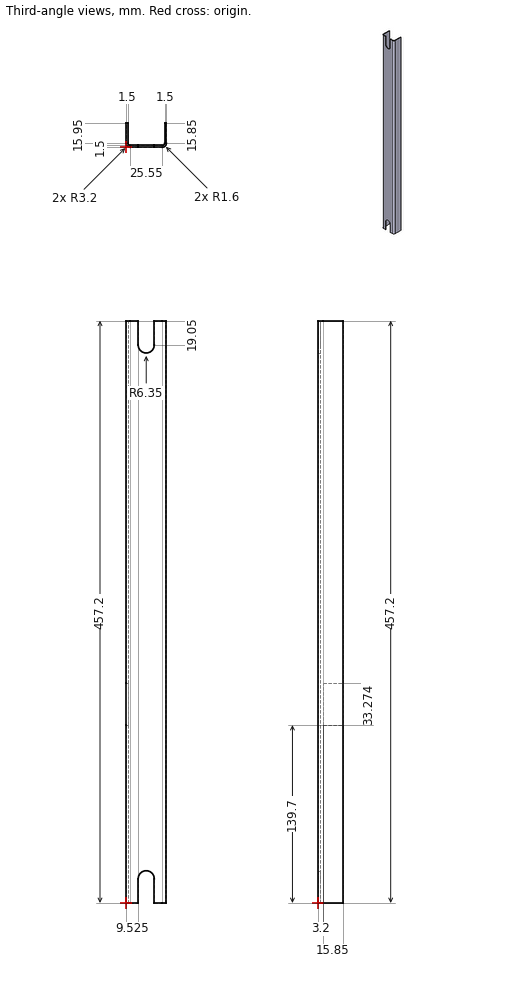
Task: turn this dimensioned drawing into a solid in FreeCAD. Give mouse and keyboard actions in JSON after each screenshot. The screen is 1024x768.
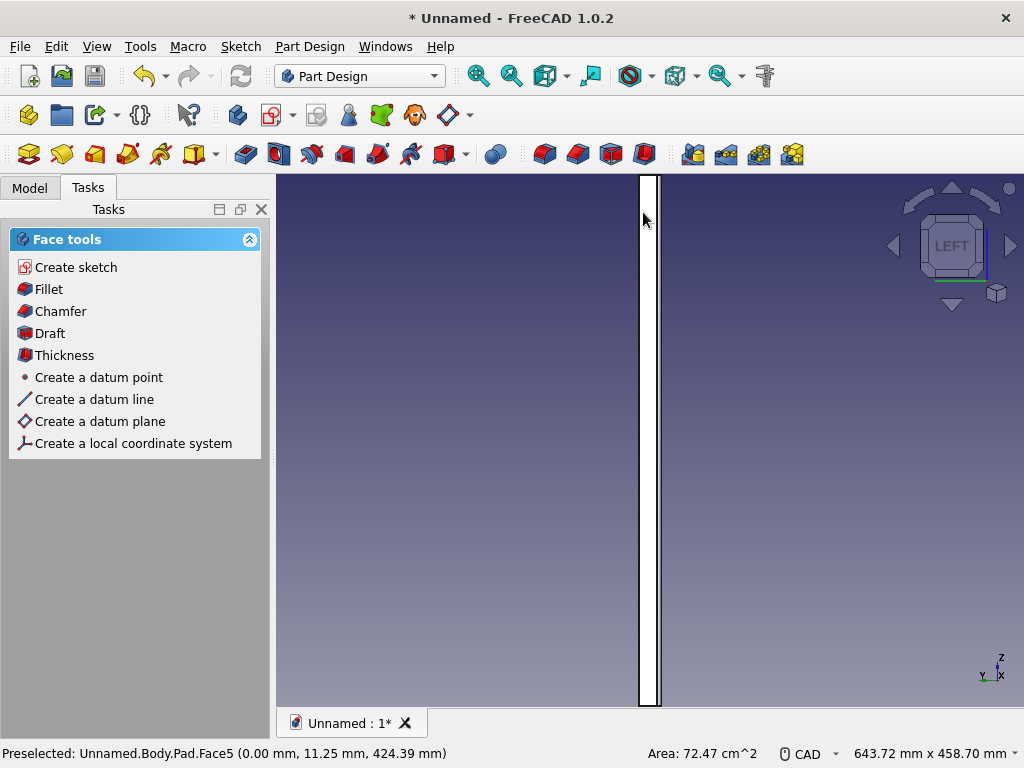
{"action": "left_click", "coordinate": [270, 116]}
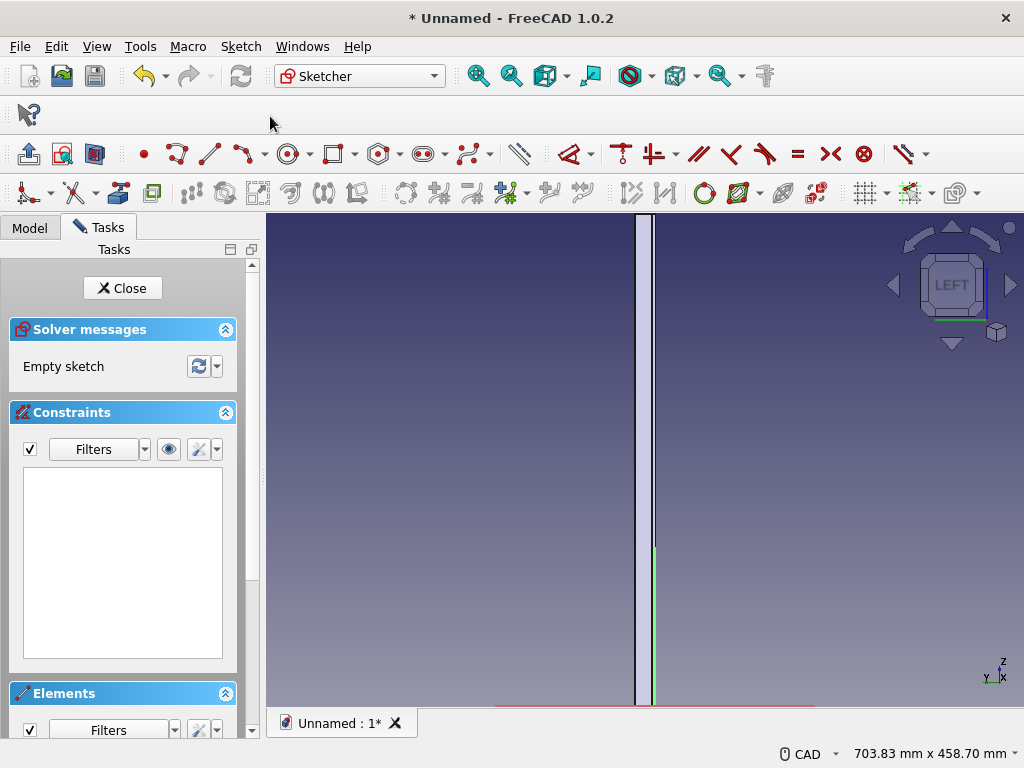
{"action": "scroll", "coordinate": [652, 548], "scroll_direction": "up", "scroll_amount": 11}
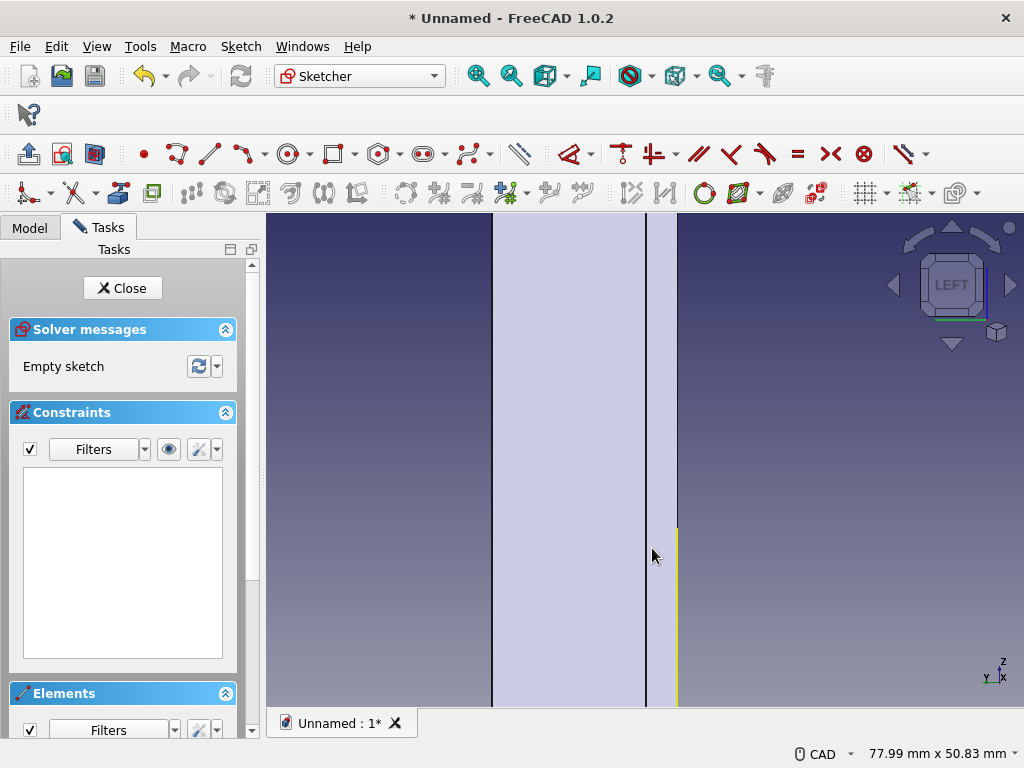
{"action": "key", "text": "g r"}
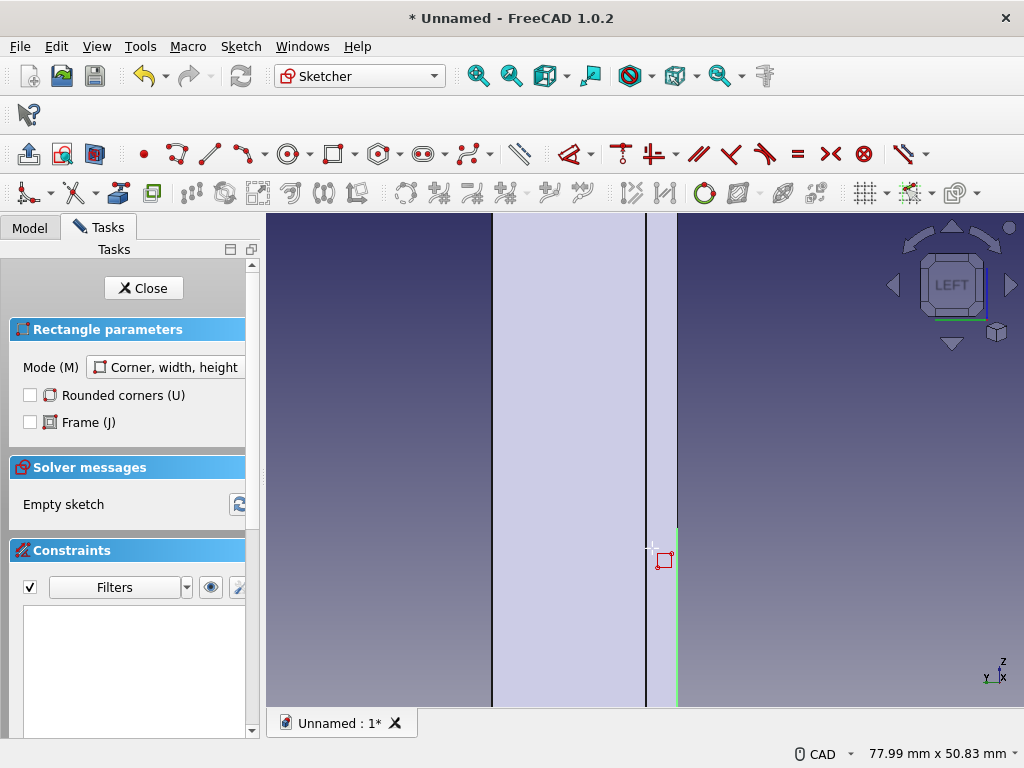
{"action": "left_click", "coordinate": [492, 289]}
{"action": "left_click", "coordinate": [646, 612]}
{"action": "key", "text": "Escape"}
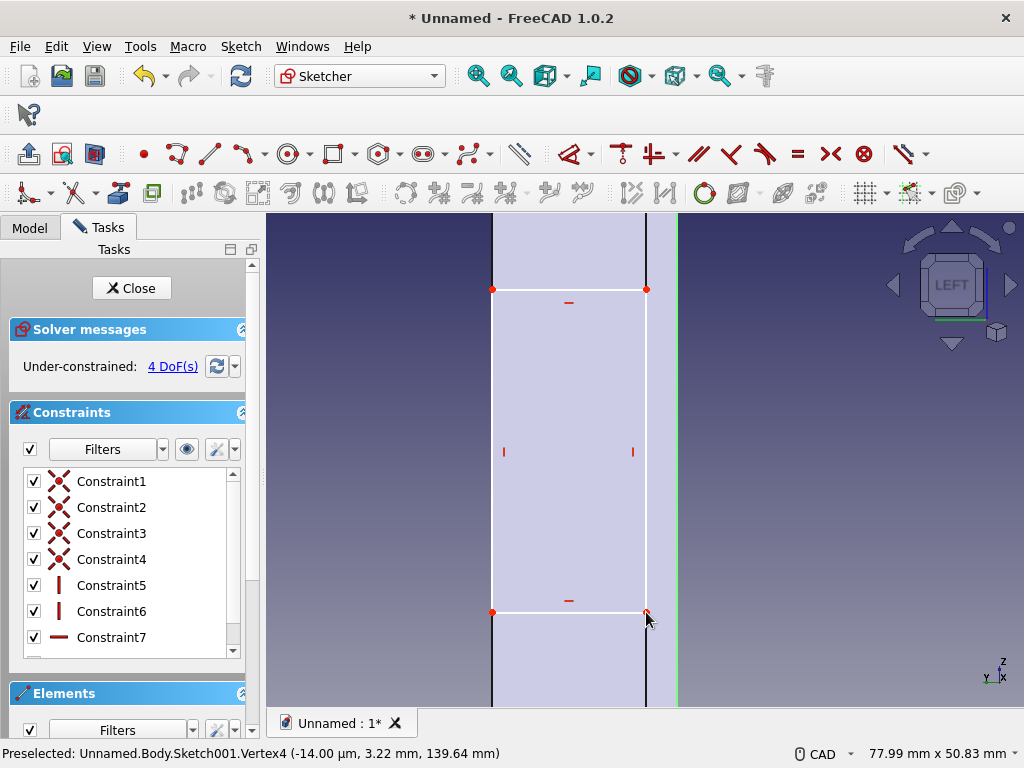
{"action": "key", "text": "d"}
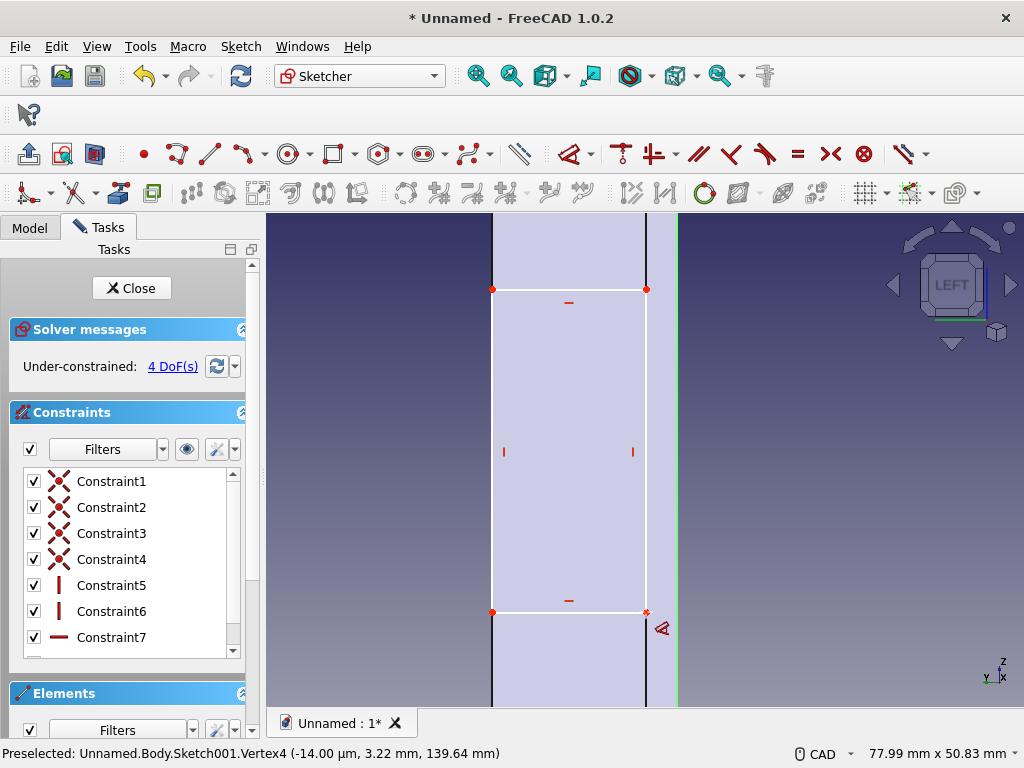
{"action": "scroll", "coordinate": [646, 613], "scroll_direction": "up", "scroll_amount": 2}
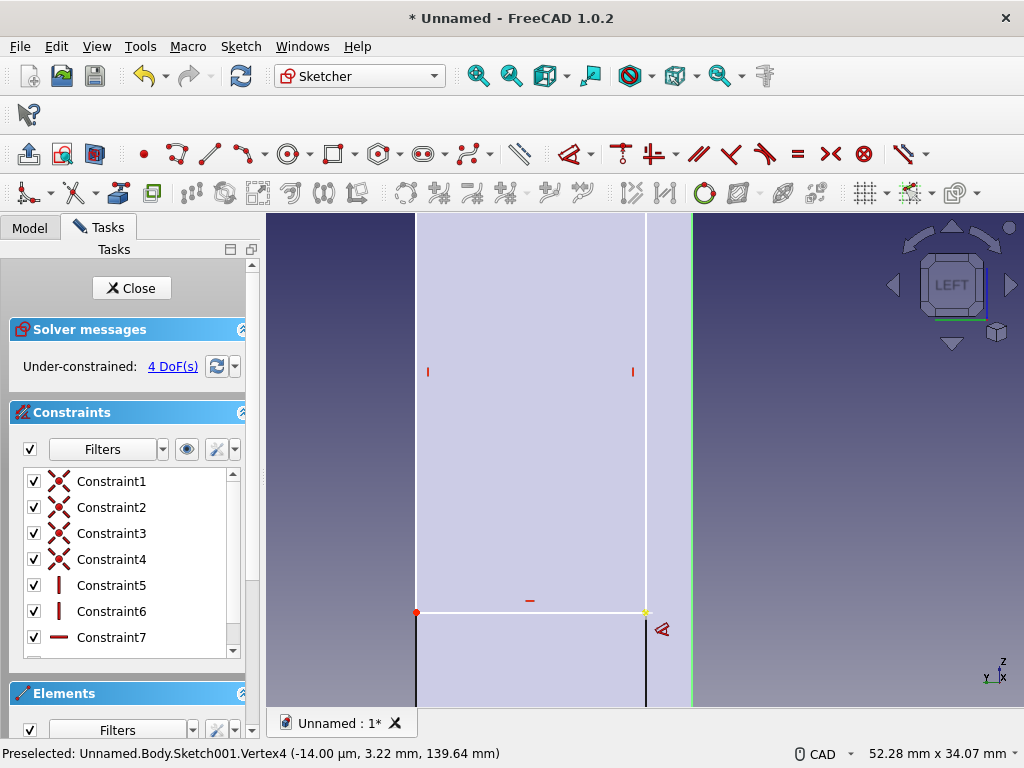
{"action": "left_click", "coordinate": [646, 613]}
{"action": "left_click", "coordinate": [669, 579]}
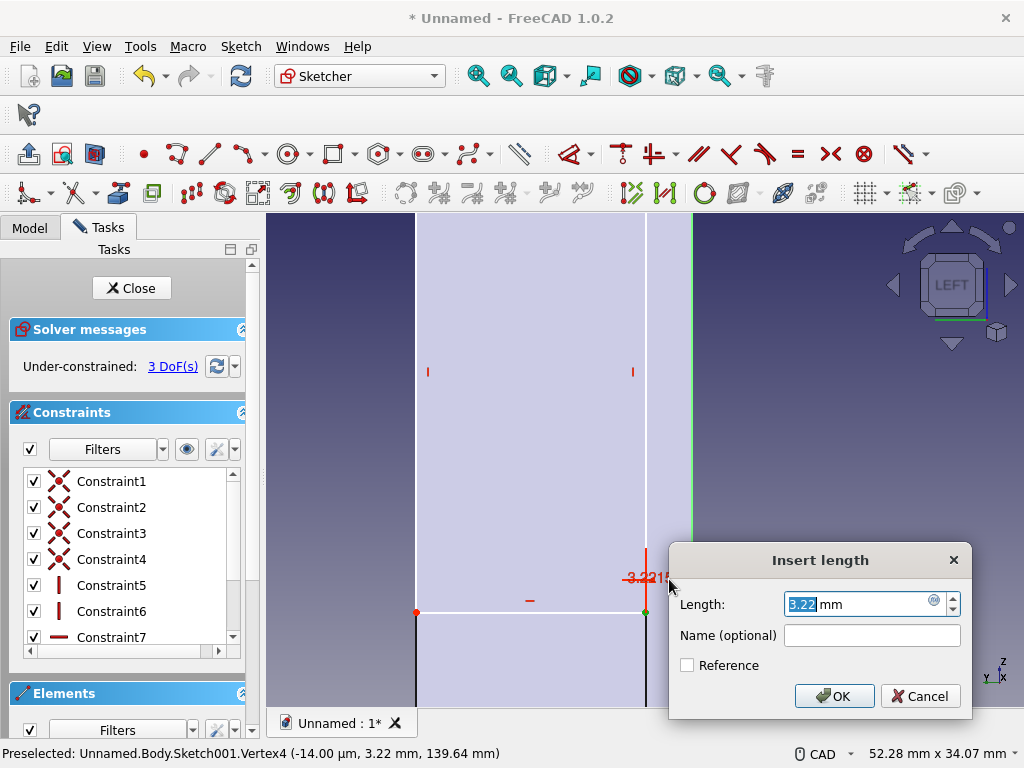
{"action": "type", "text": "3.2"}
{"action": "key", "text": "Return"}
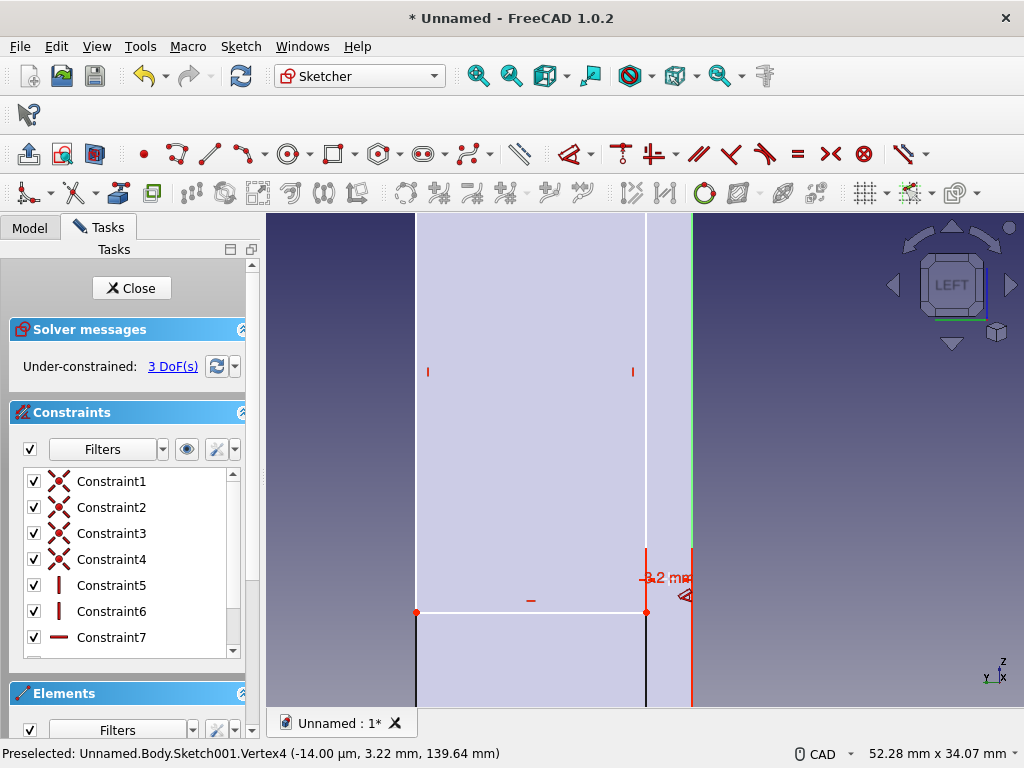
{"action": "left_click", "coordinate": [485, 613]}
{"action": "left_click", "coordinate": [531, 647]}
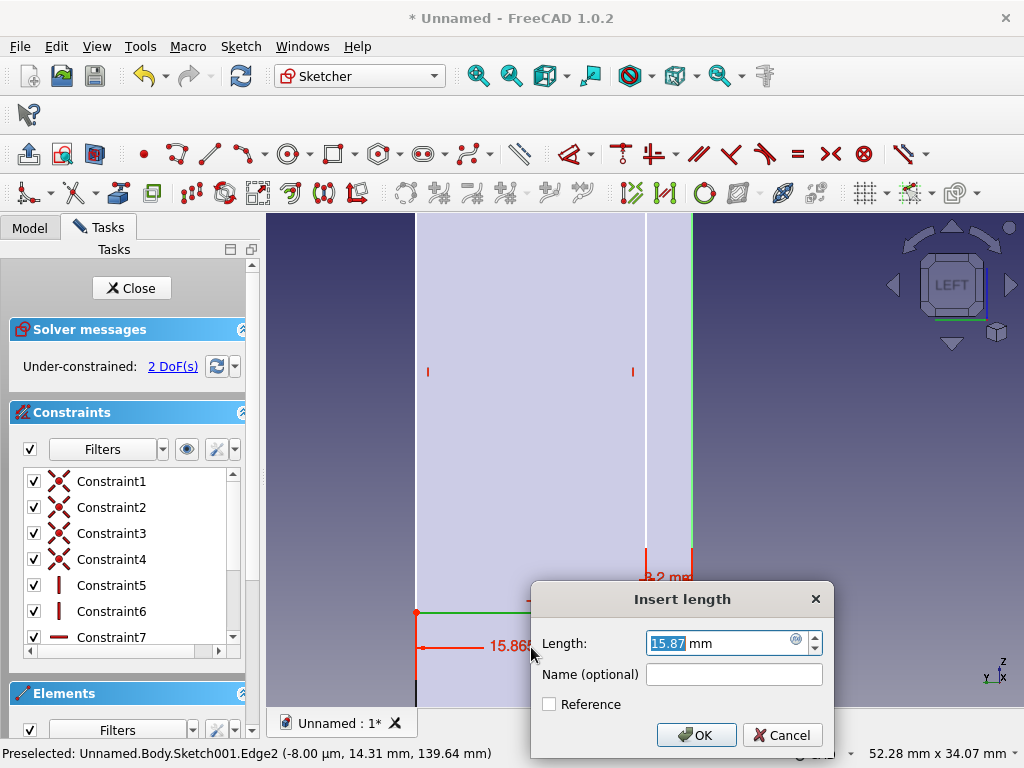
{"action": "type", "text": "15.85"}
{"action": "key", "text": "Return"}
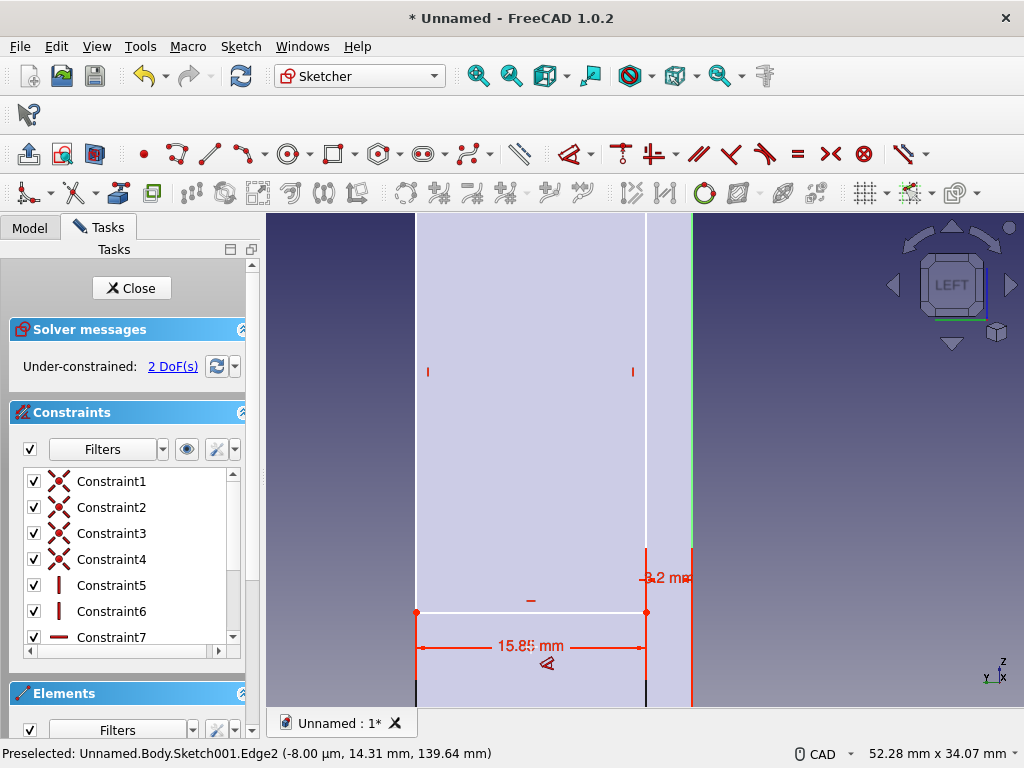
{"action": "left_click", "coordinate": [416, 275]}
{"action": "left_click", "coordinate": [382, 427]}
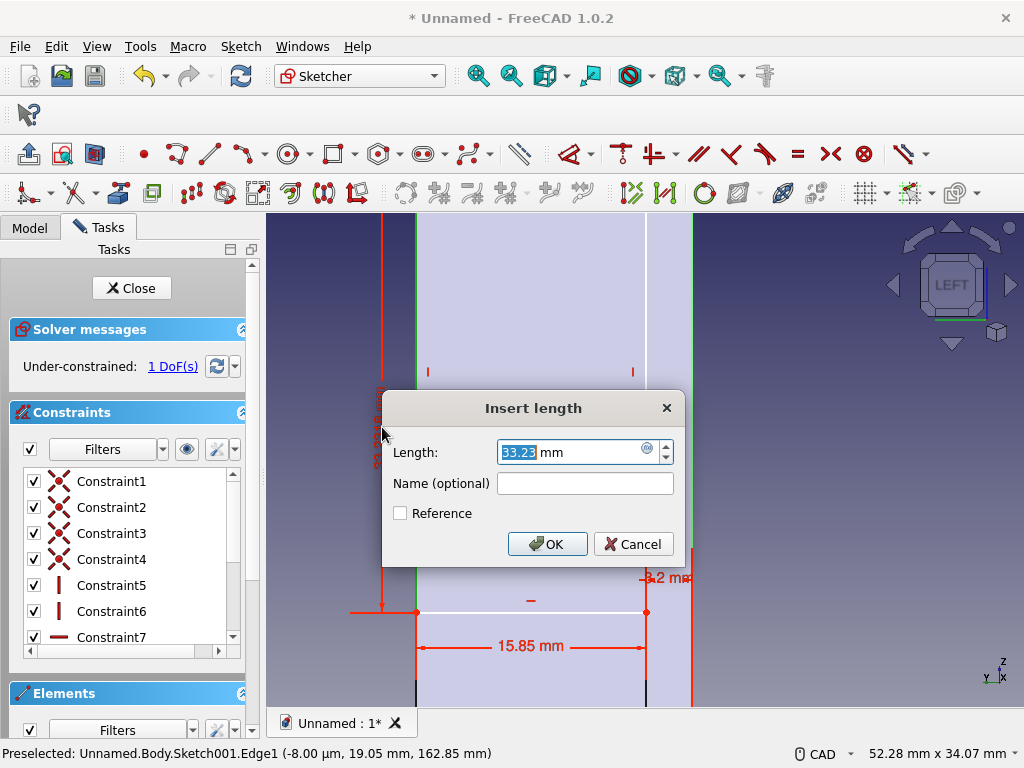
{"action": "type", "text": "33.274"}
{"action": "key", "text": "Return"}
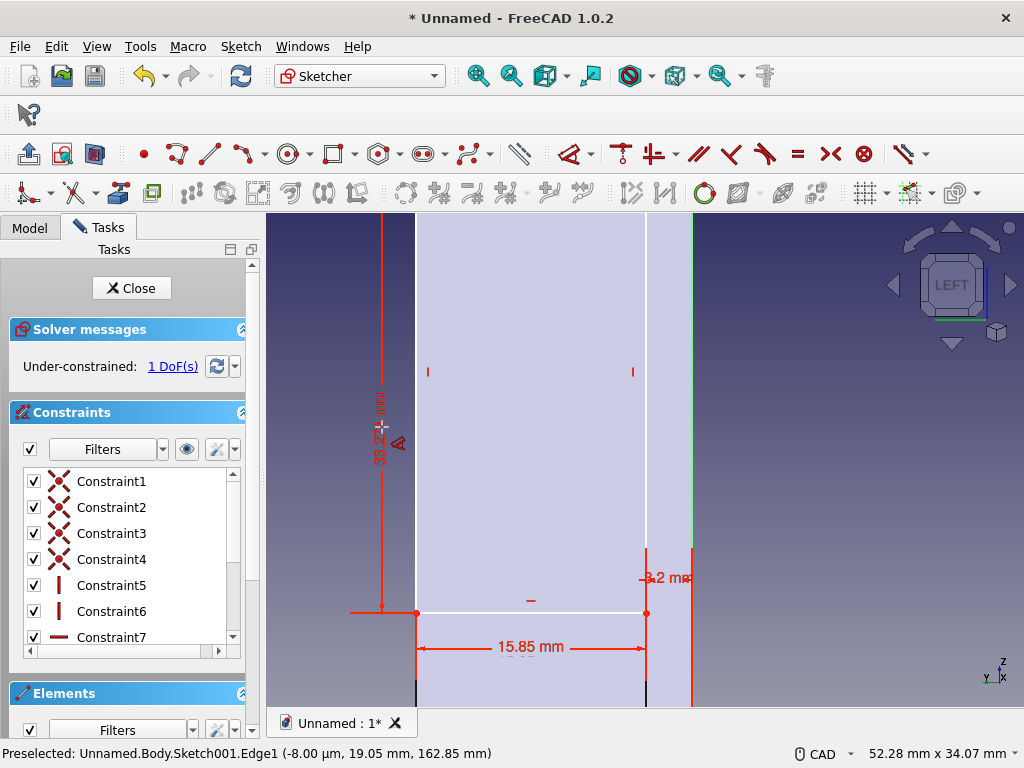
{"action": "left_click", "coordinate": [416, 613]}
{"action": "left_click", "coordinate": [726, 646]}